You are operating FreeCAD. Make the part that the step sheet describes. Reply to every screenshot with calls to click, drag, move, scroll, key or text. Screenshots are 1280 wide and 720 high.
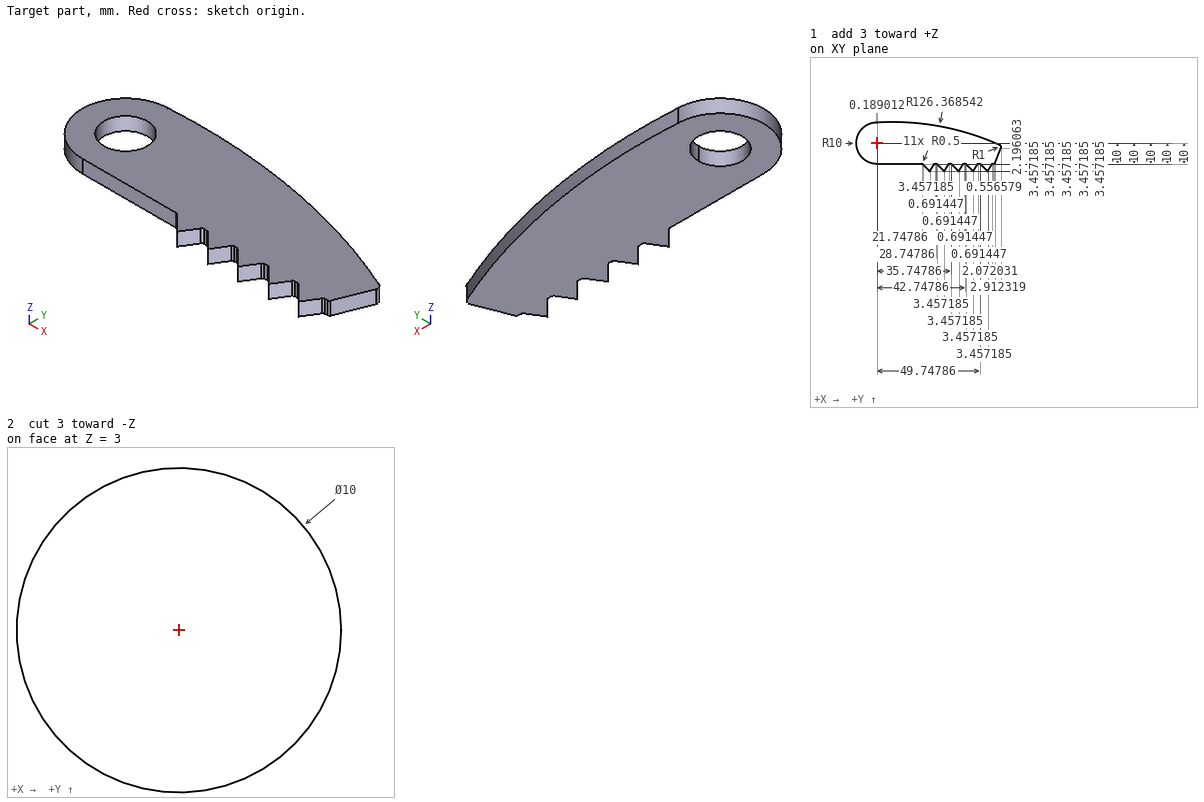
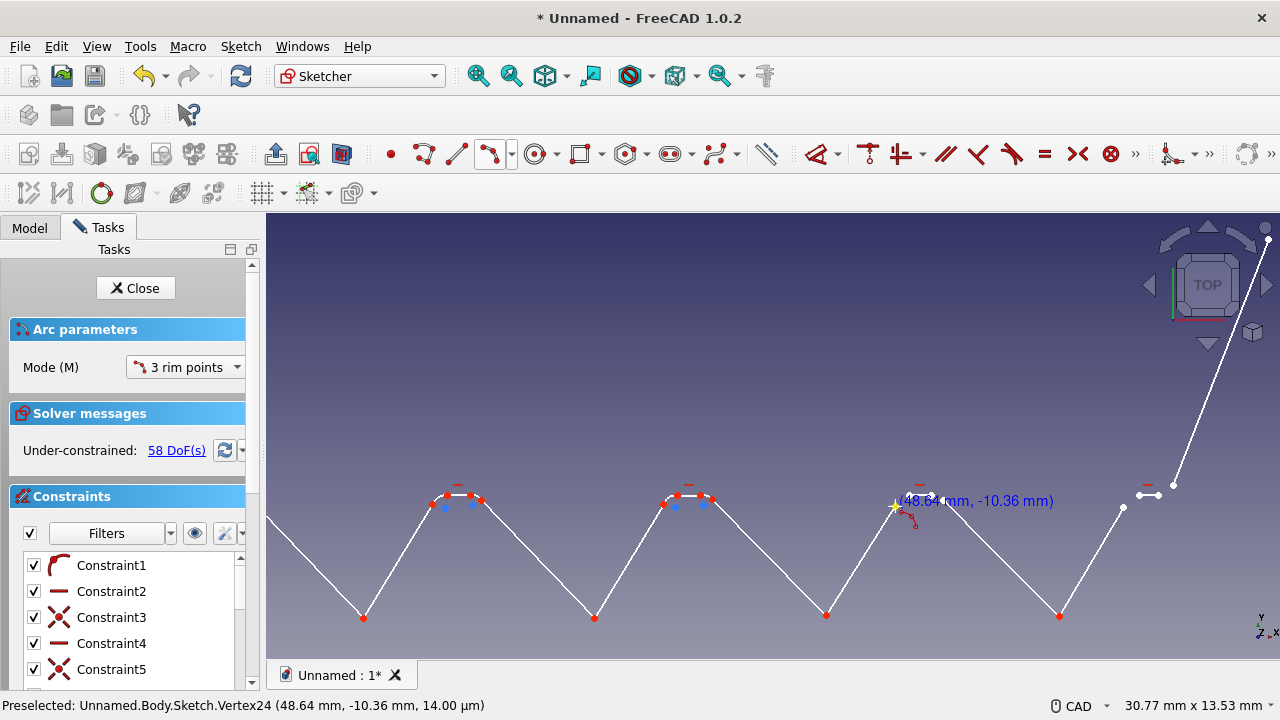
scroll(909, 494, up, 2)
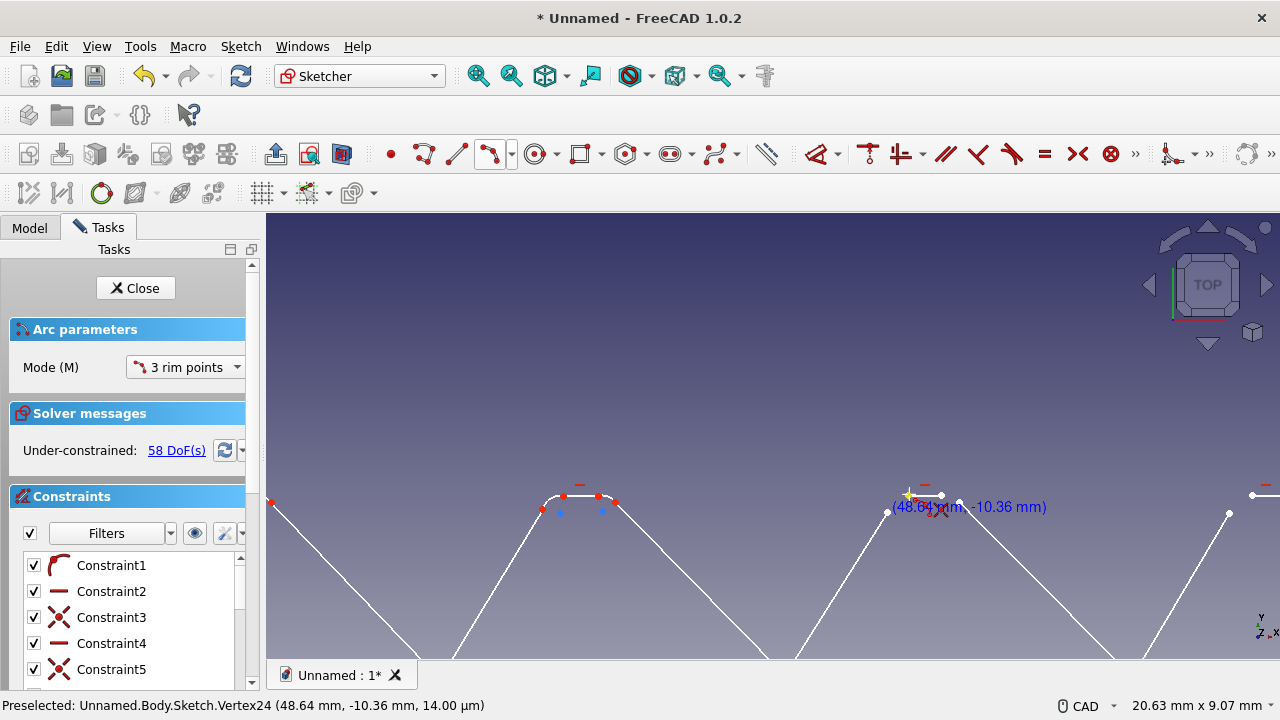
click(909, 496)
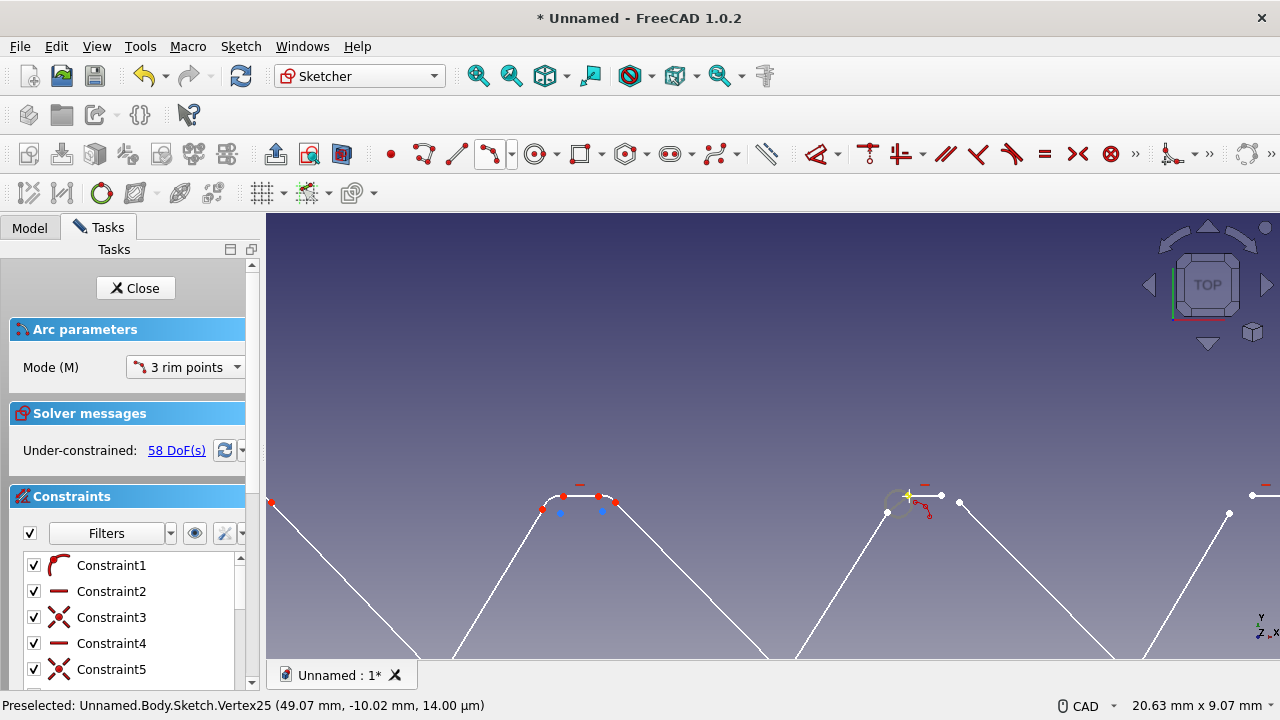
scroll(896, 497, up, 9)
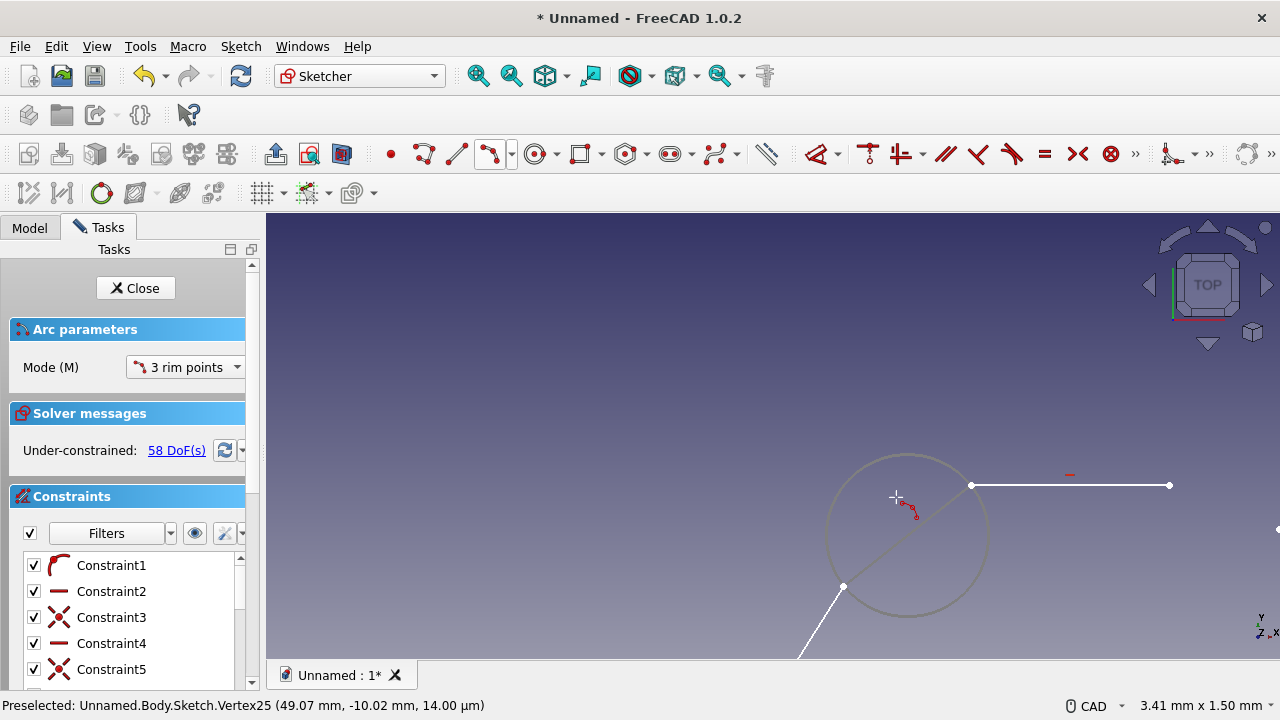
click(896, 497)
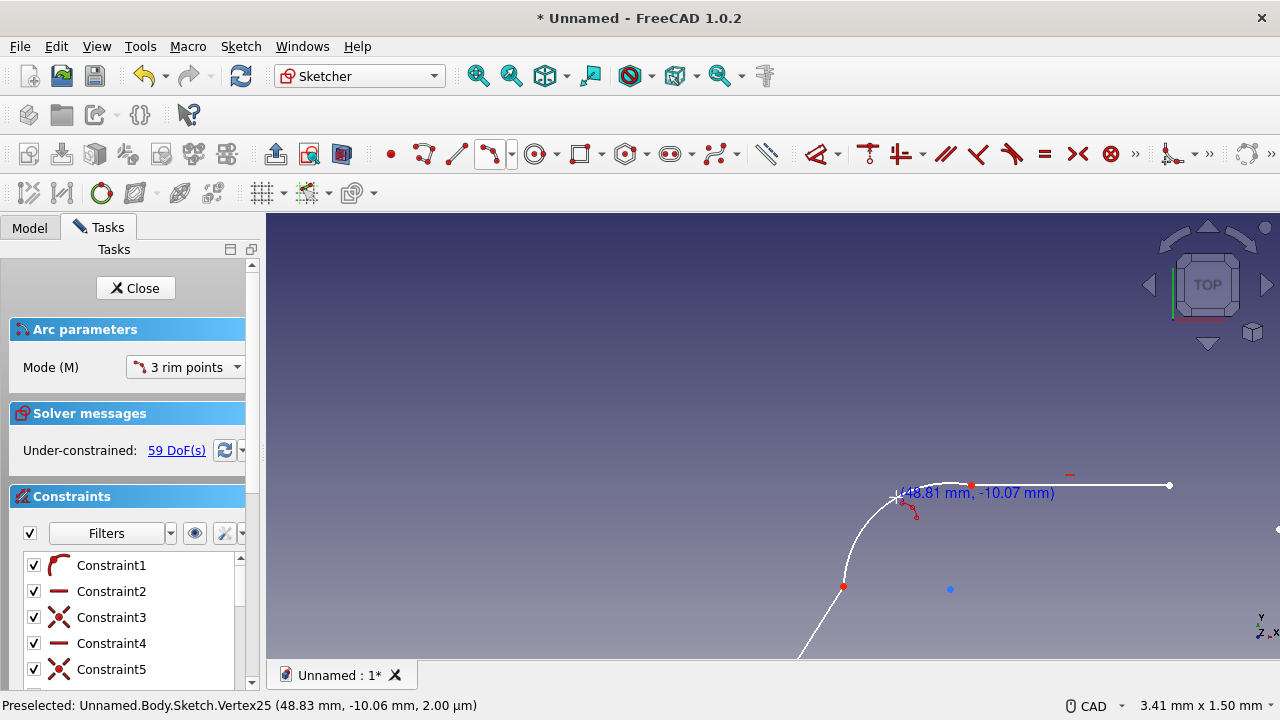
scroll(942, 519, down, 17)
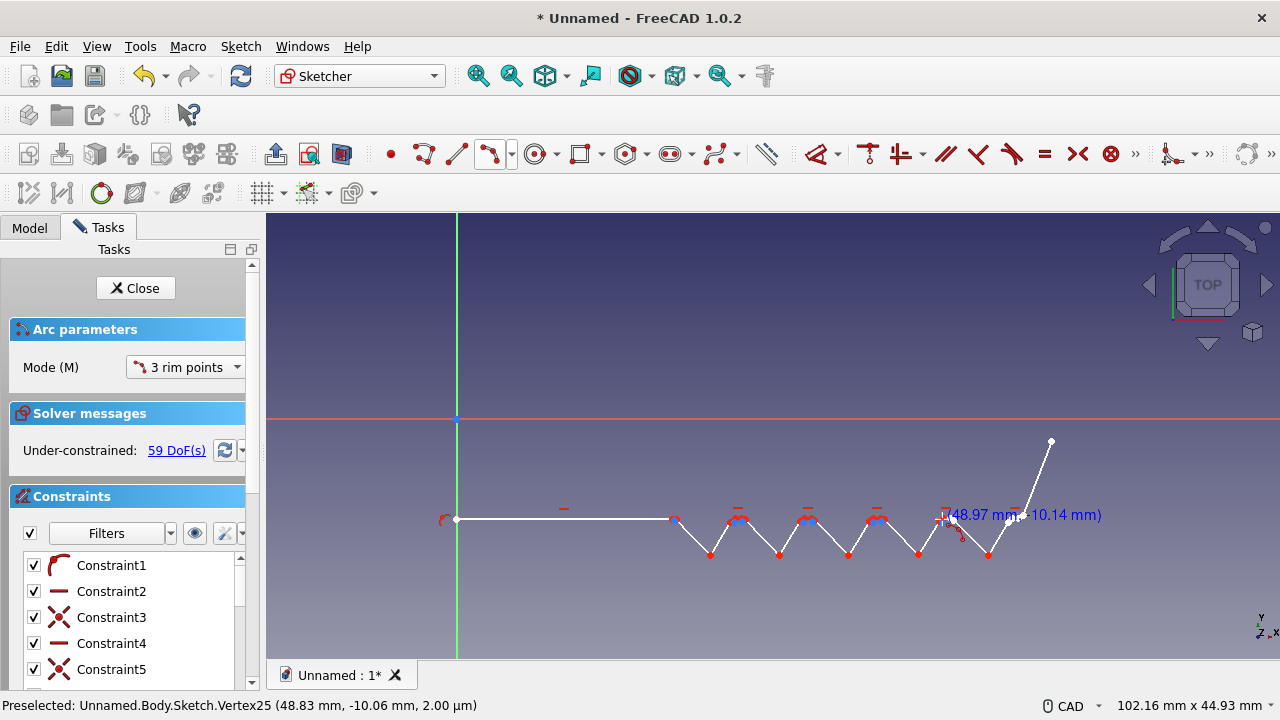
scroll(950, 518, up, 8)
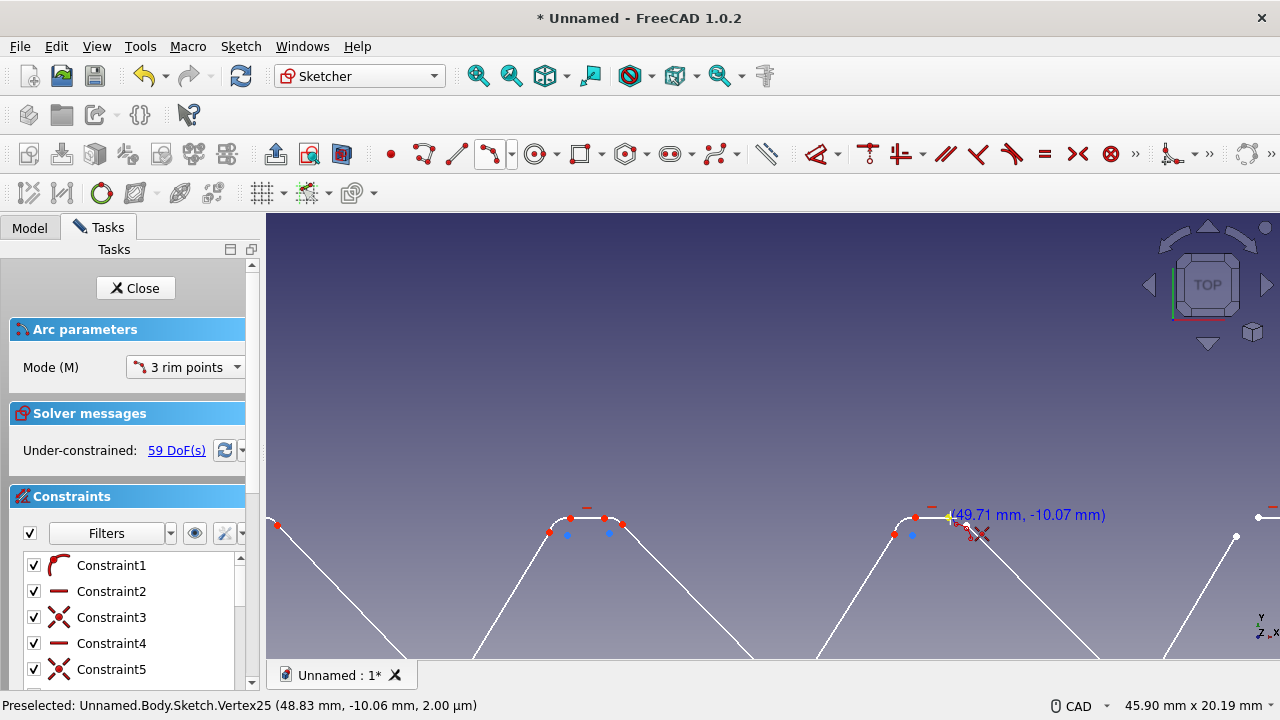
click(949, 518)
click(967, 525)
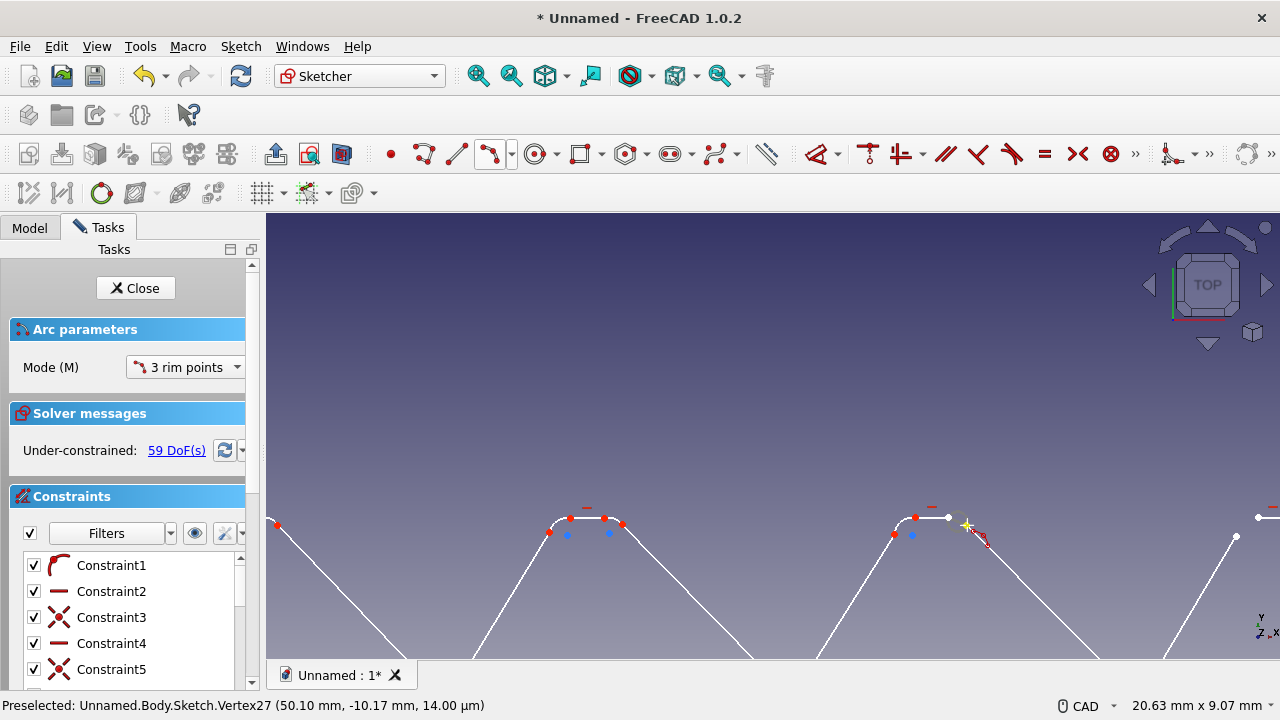
scroll(959, 519, up, 11)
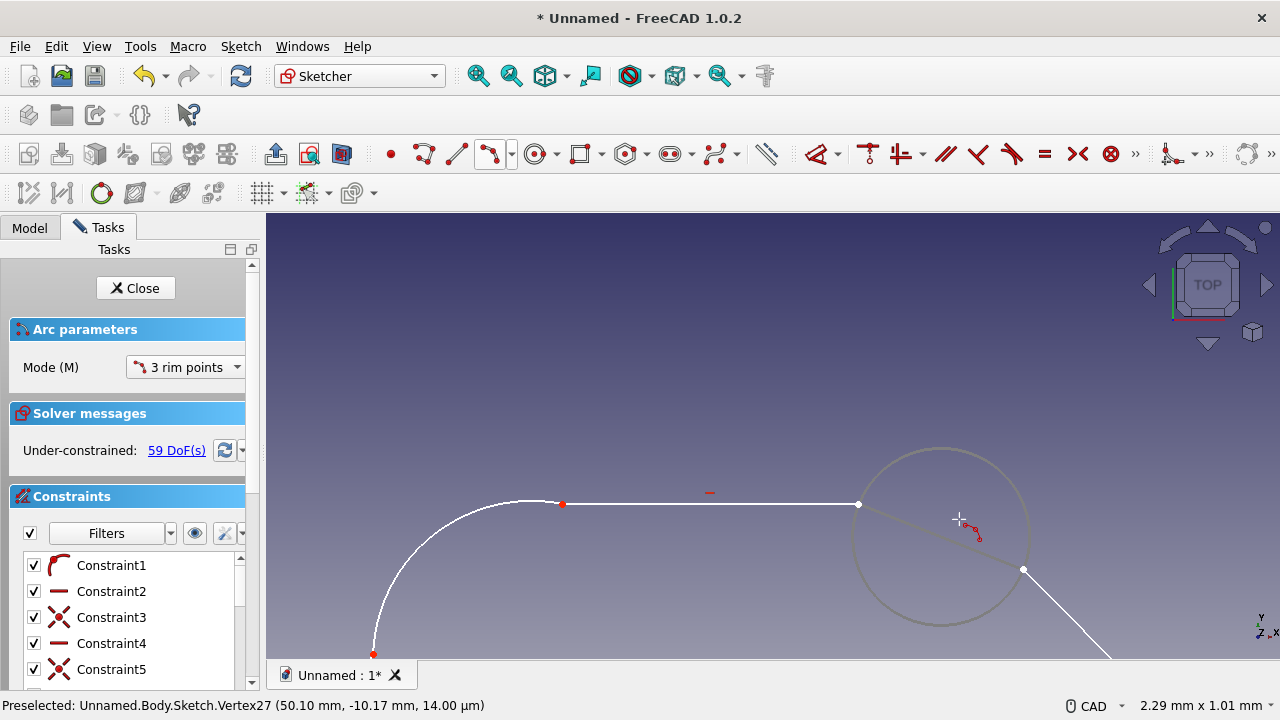
click(950, 510)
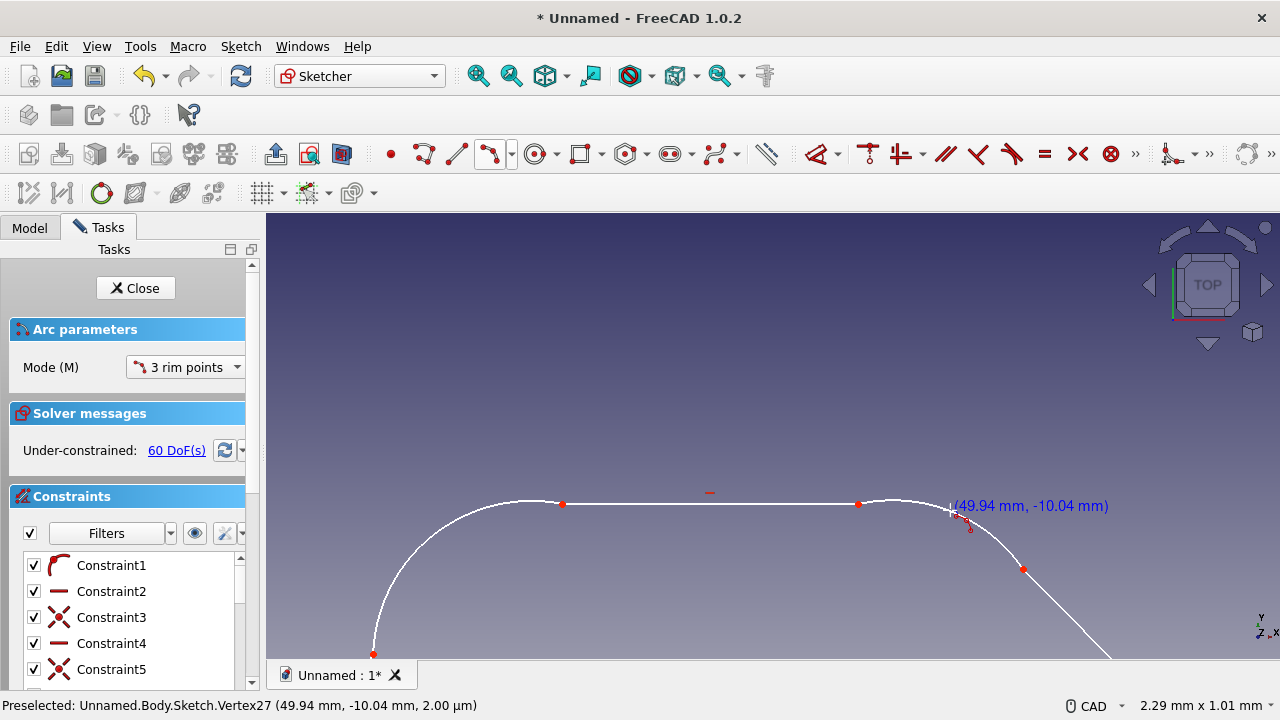
scroll(704, 436, down, 15)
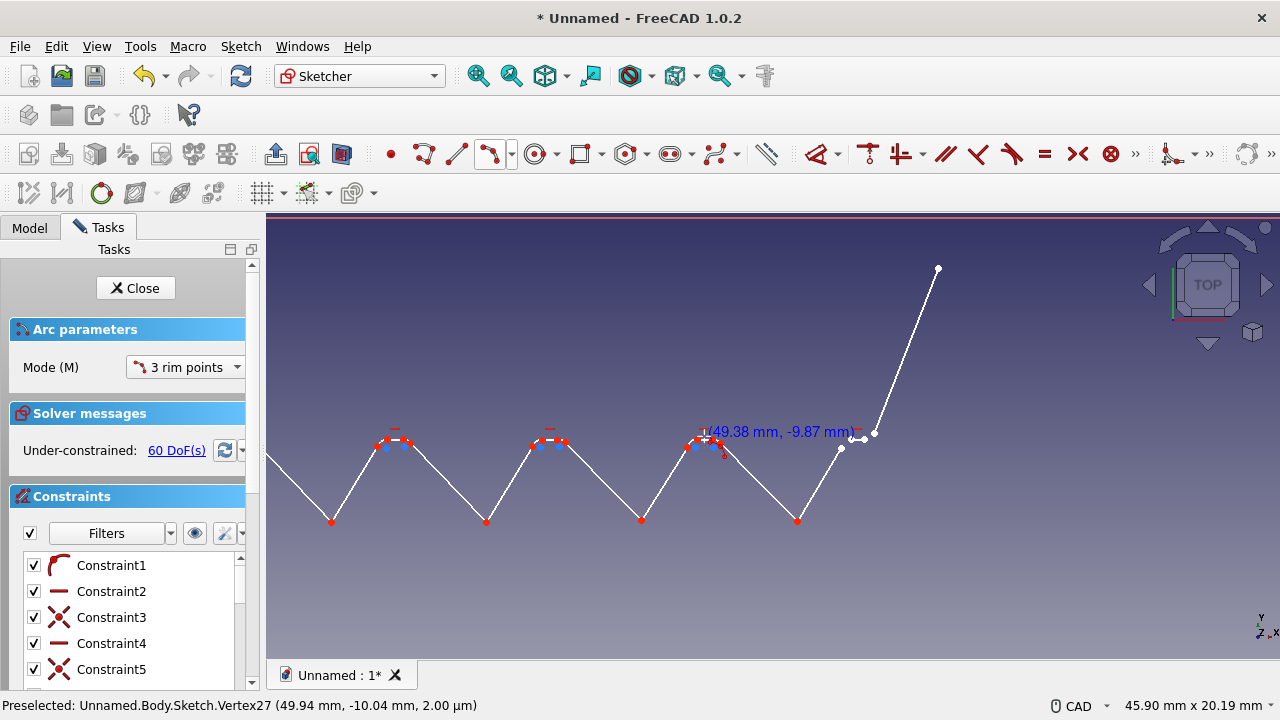
scroll(1018, 539, down, 5)